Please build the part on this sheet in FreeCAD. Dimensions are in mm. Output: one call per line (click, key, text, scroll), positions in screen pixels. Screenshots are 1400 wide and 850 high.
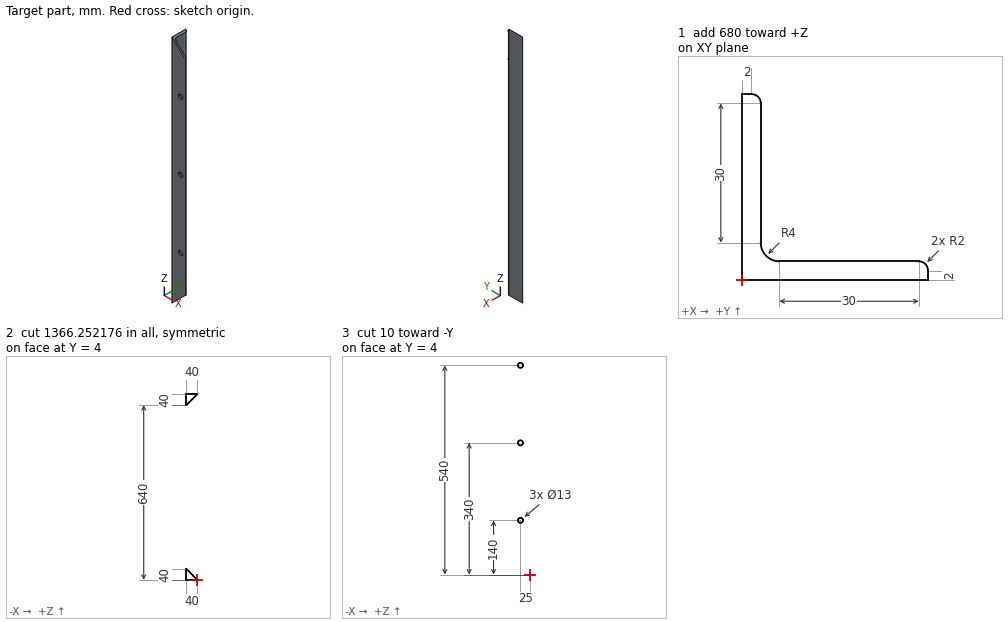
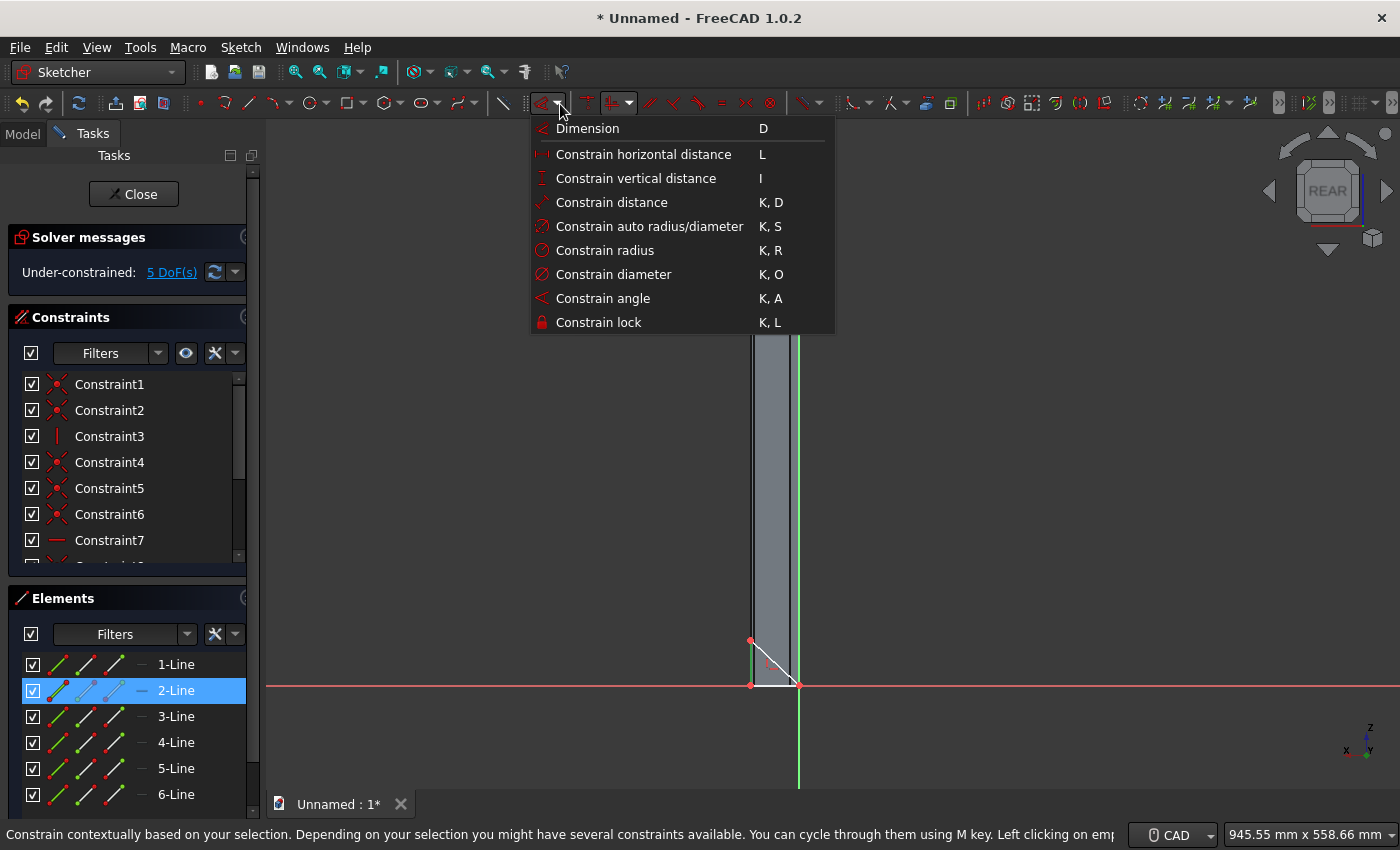
click(683, 178)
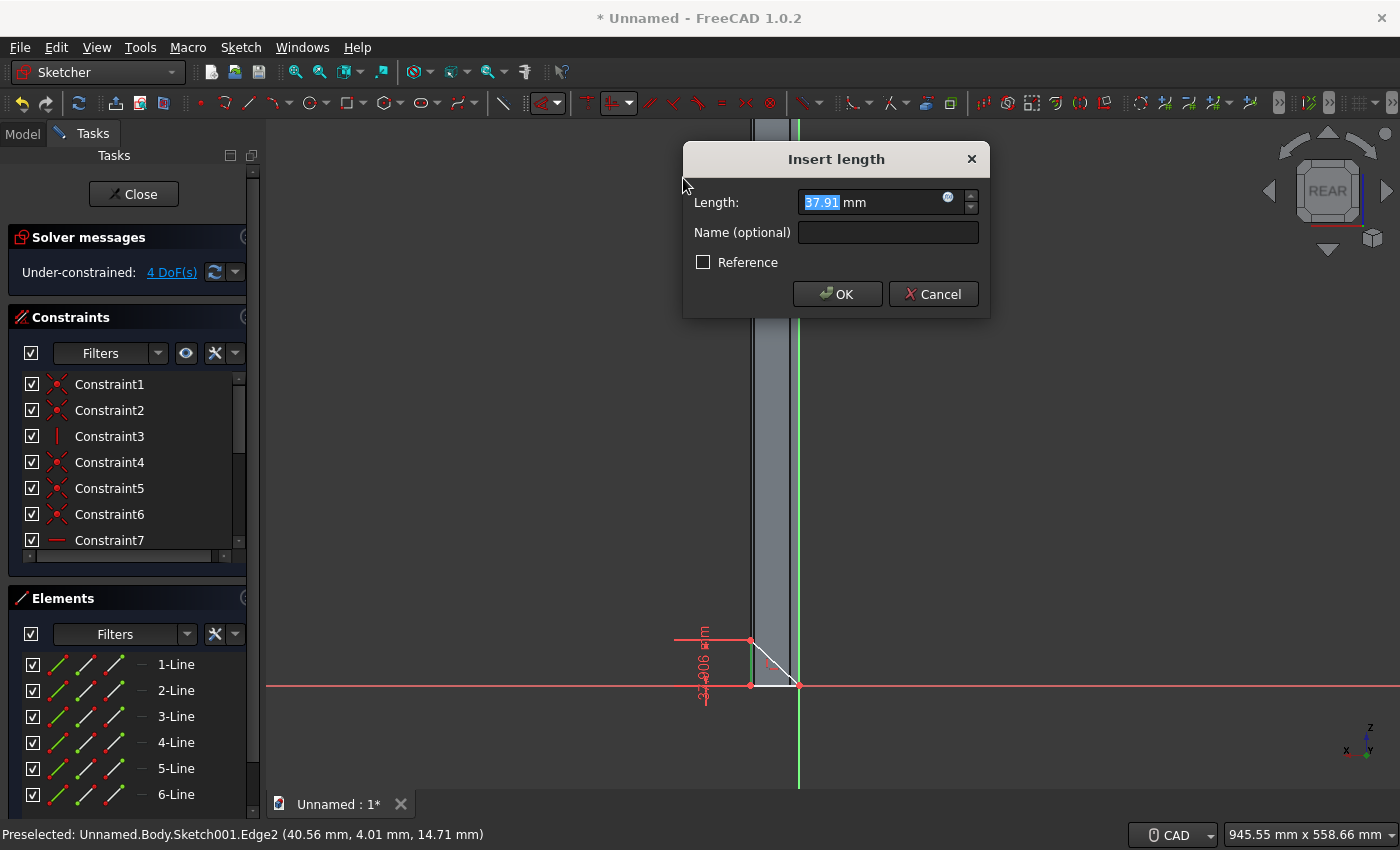
text(40)
key(Return)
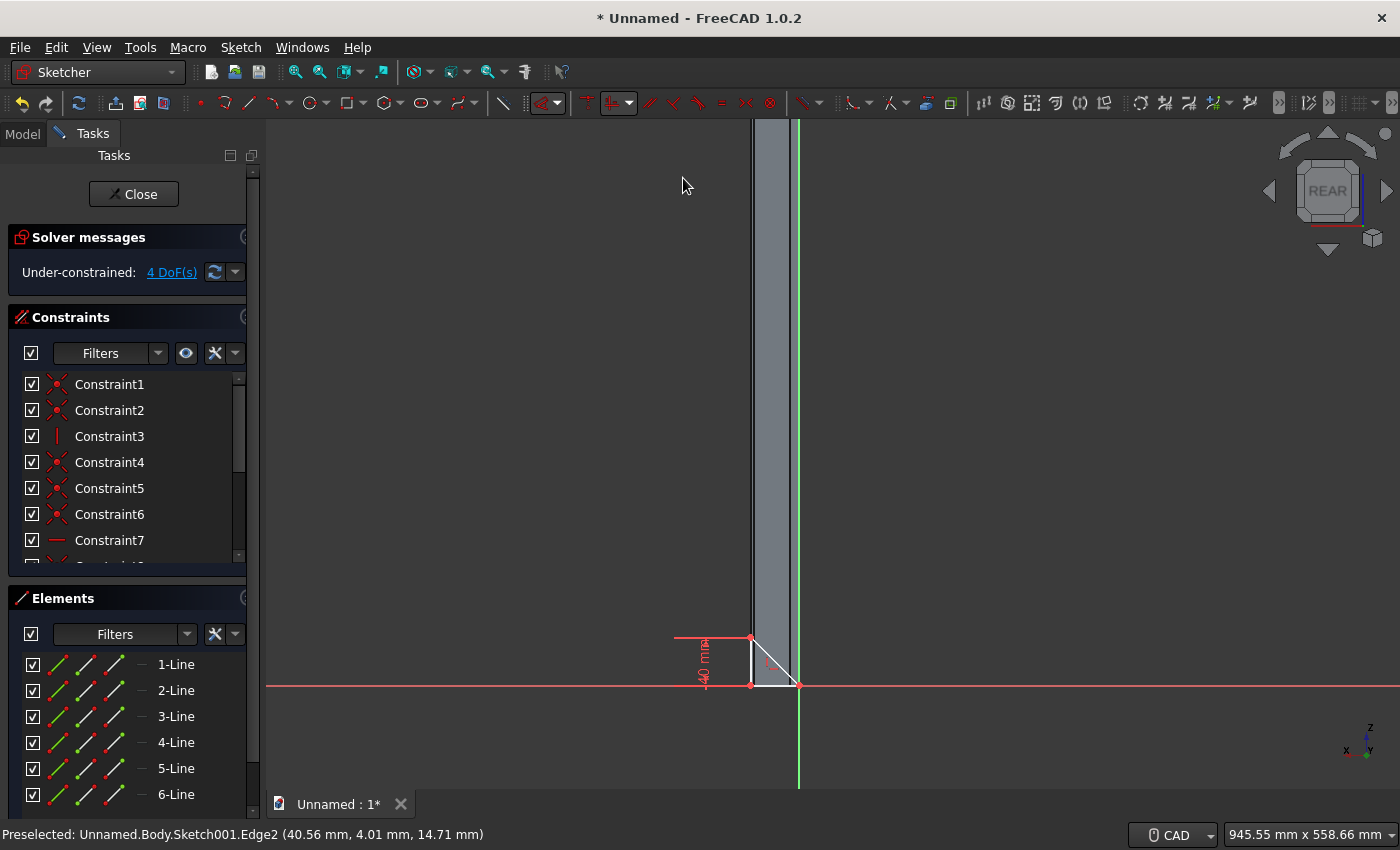
click(765, 686)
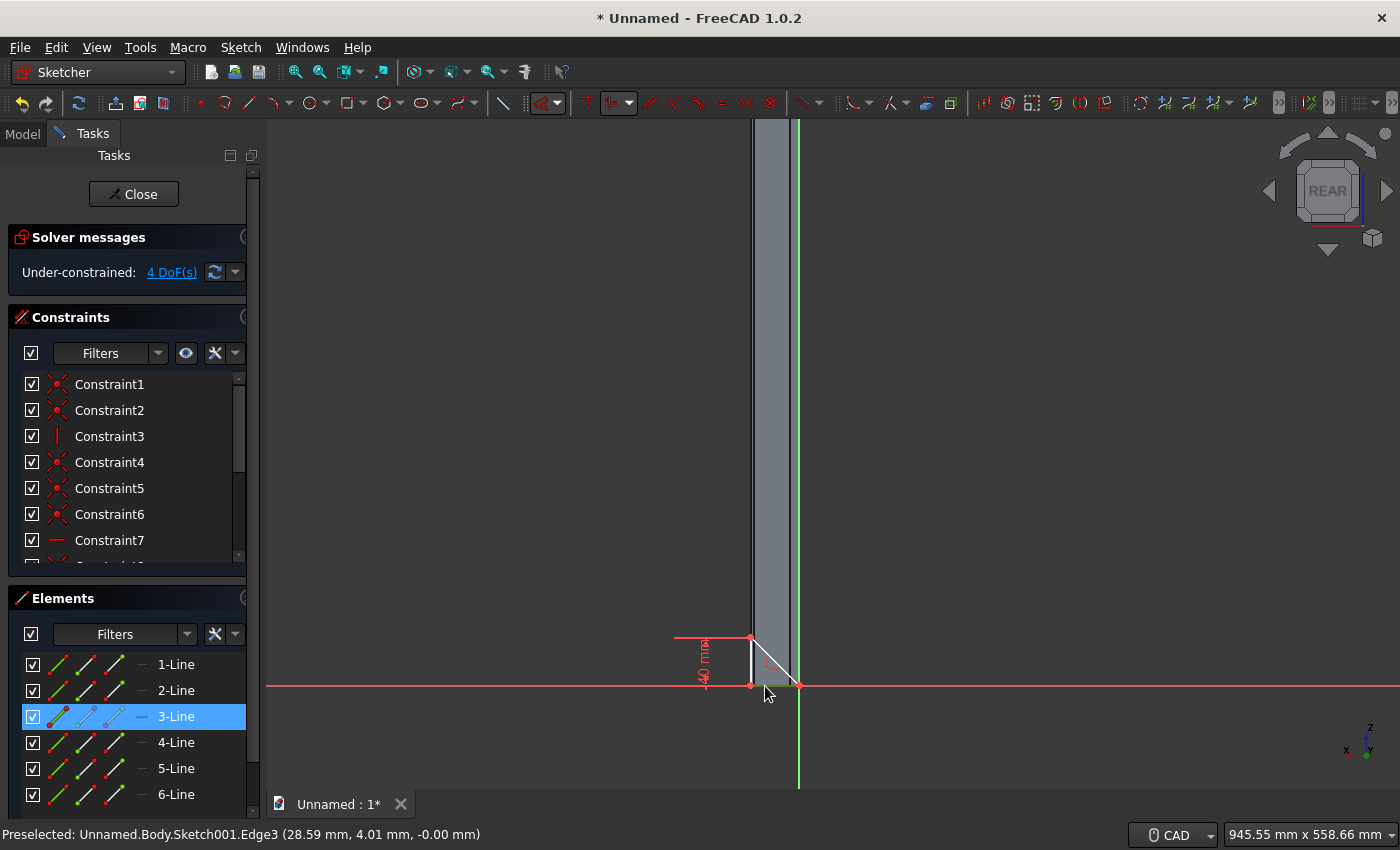
click(560, 104)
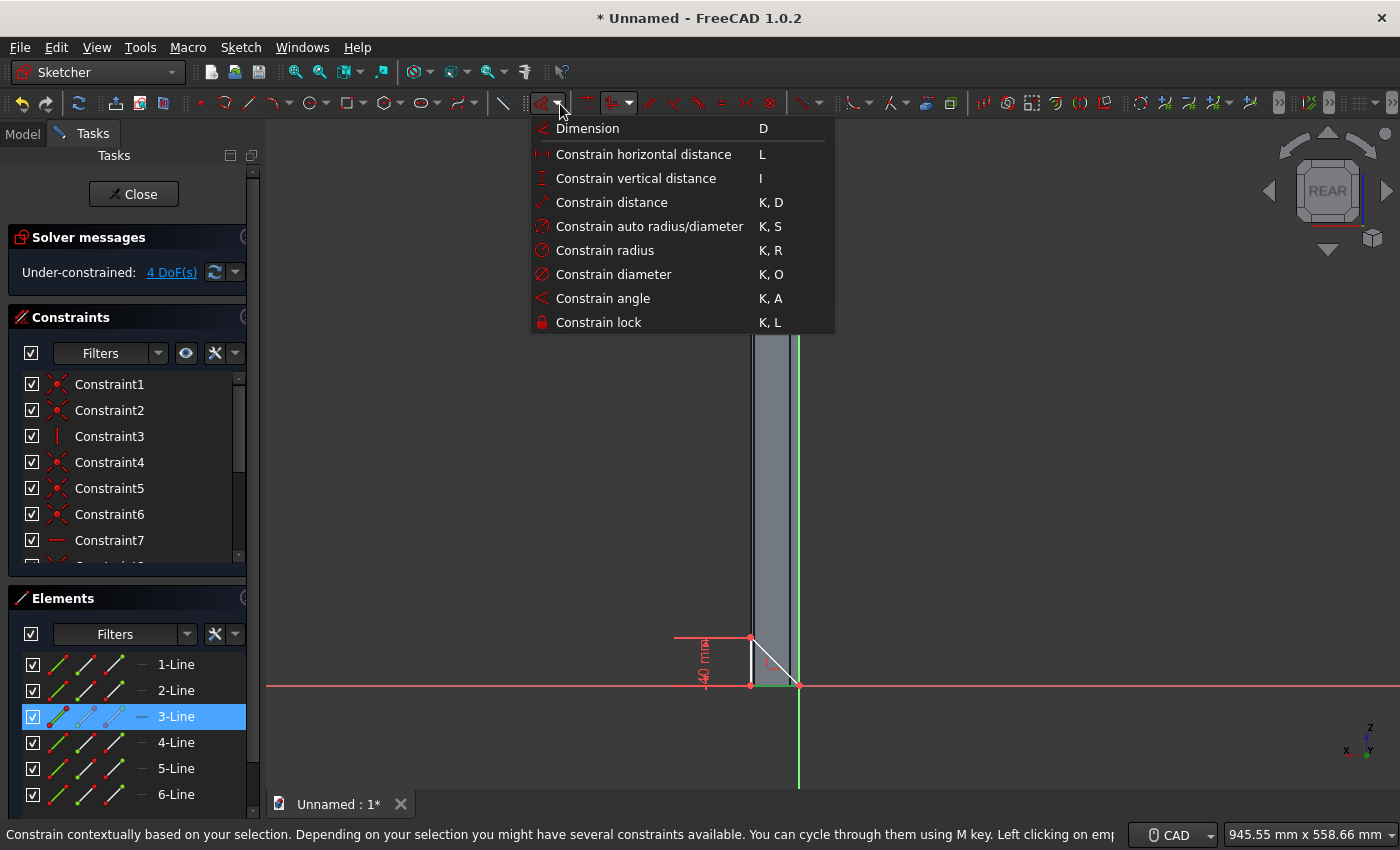
click(683, 154)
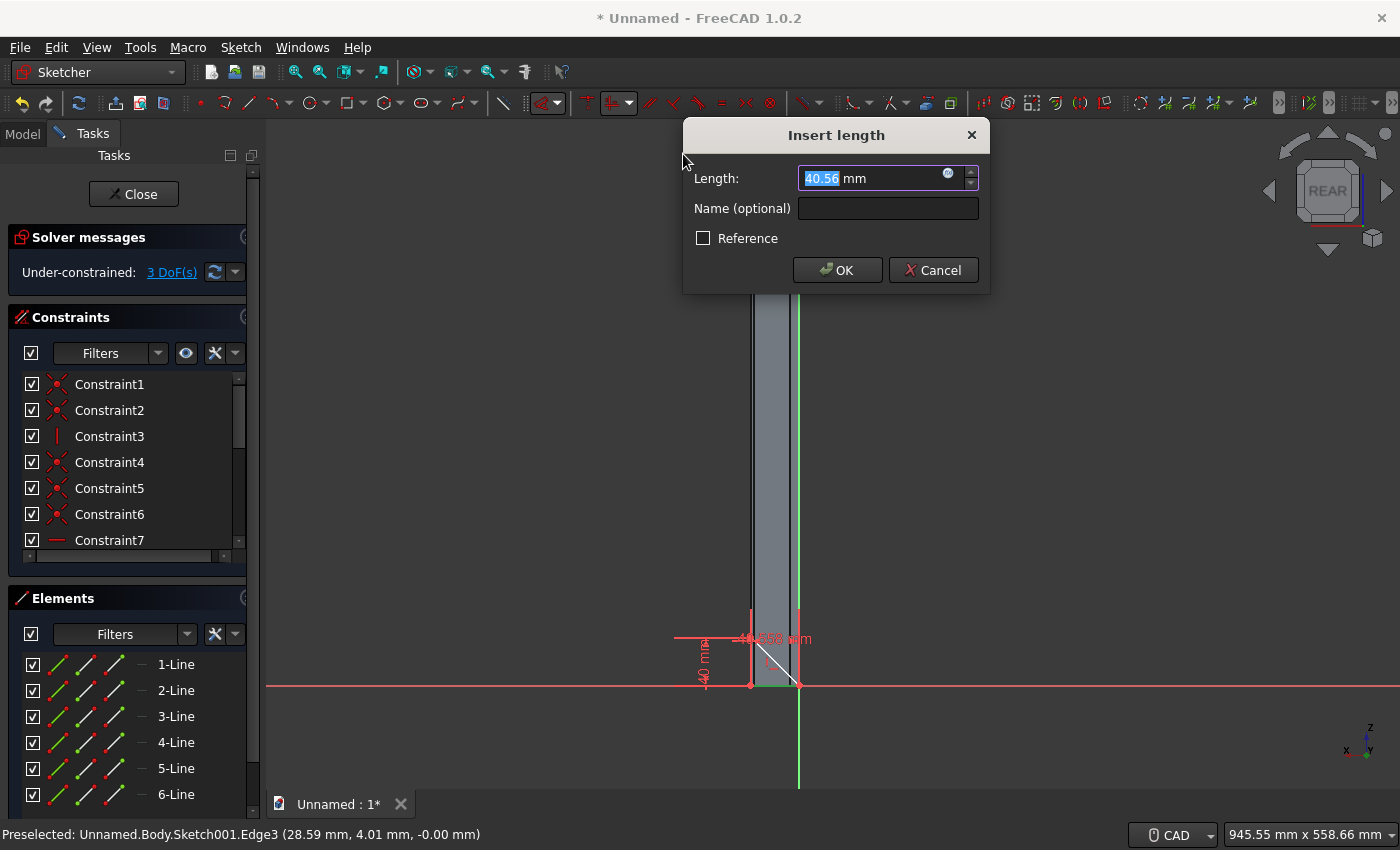
text(40)
key(Return)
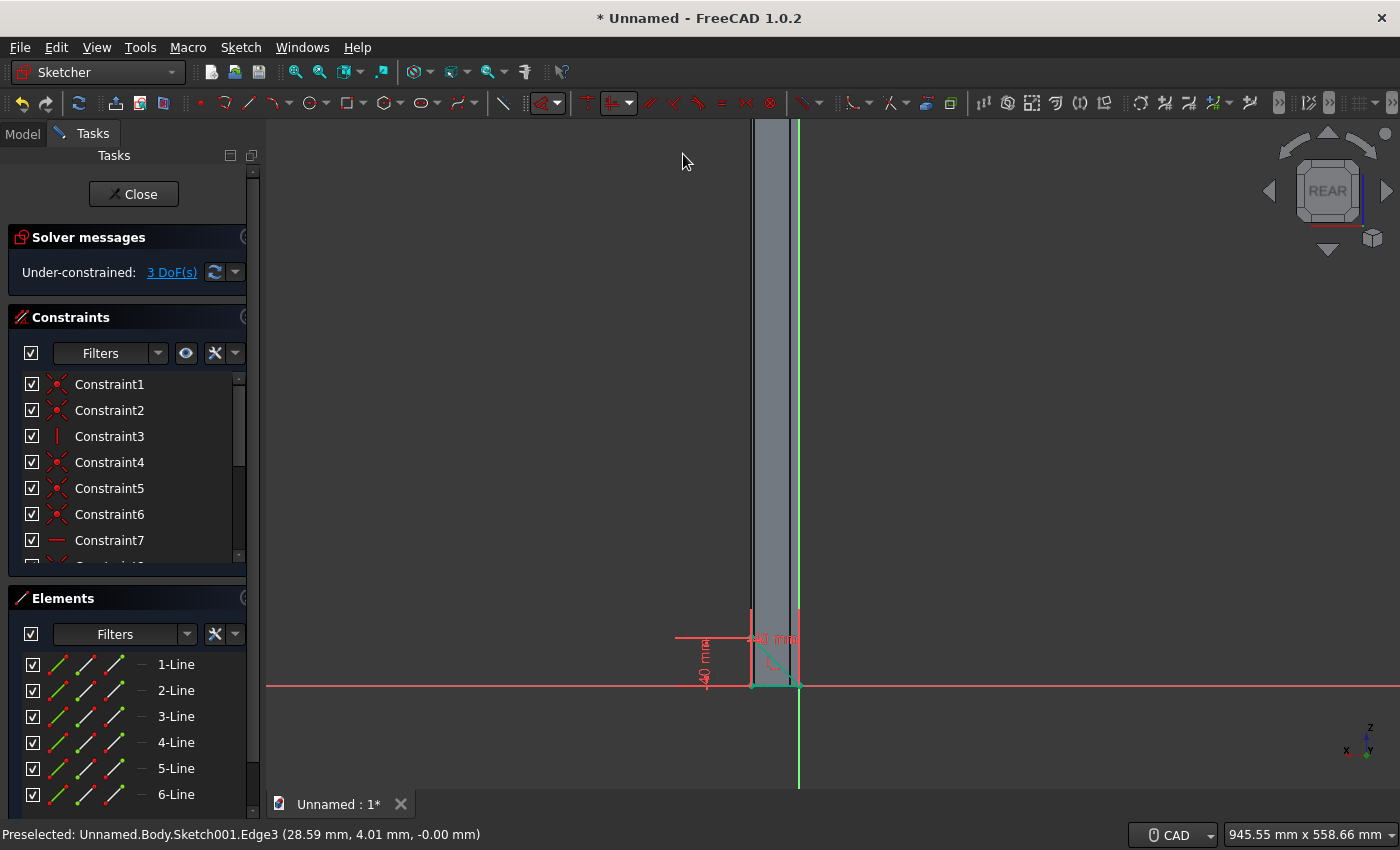
scroll(751, 668, down, 3)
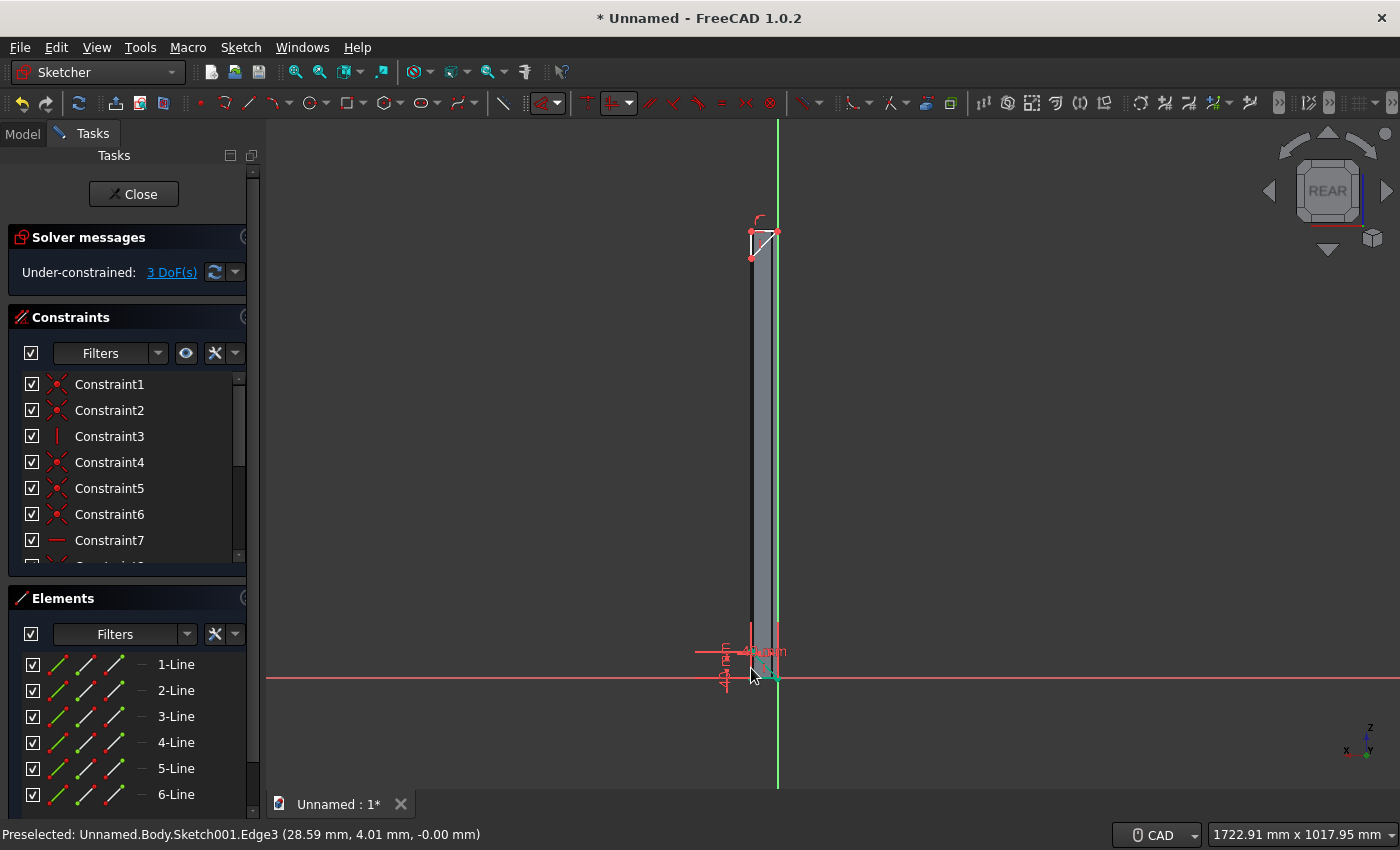
scroll(770, 231, up, 5)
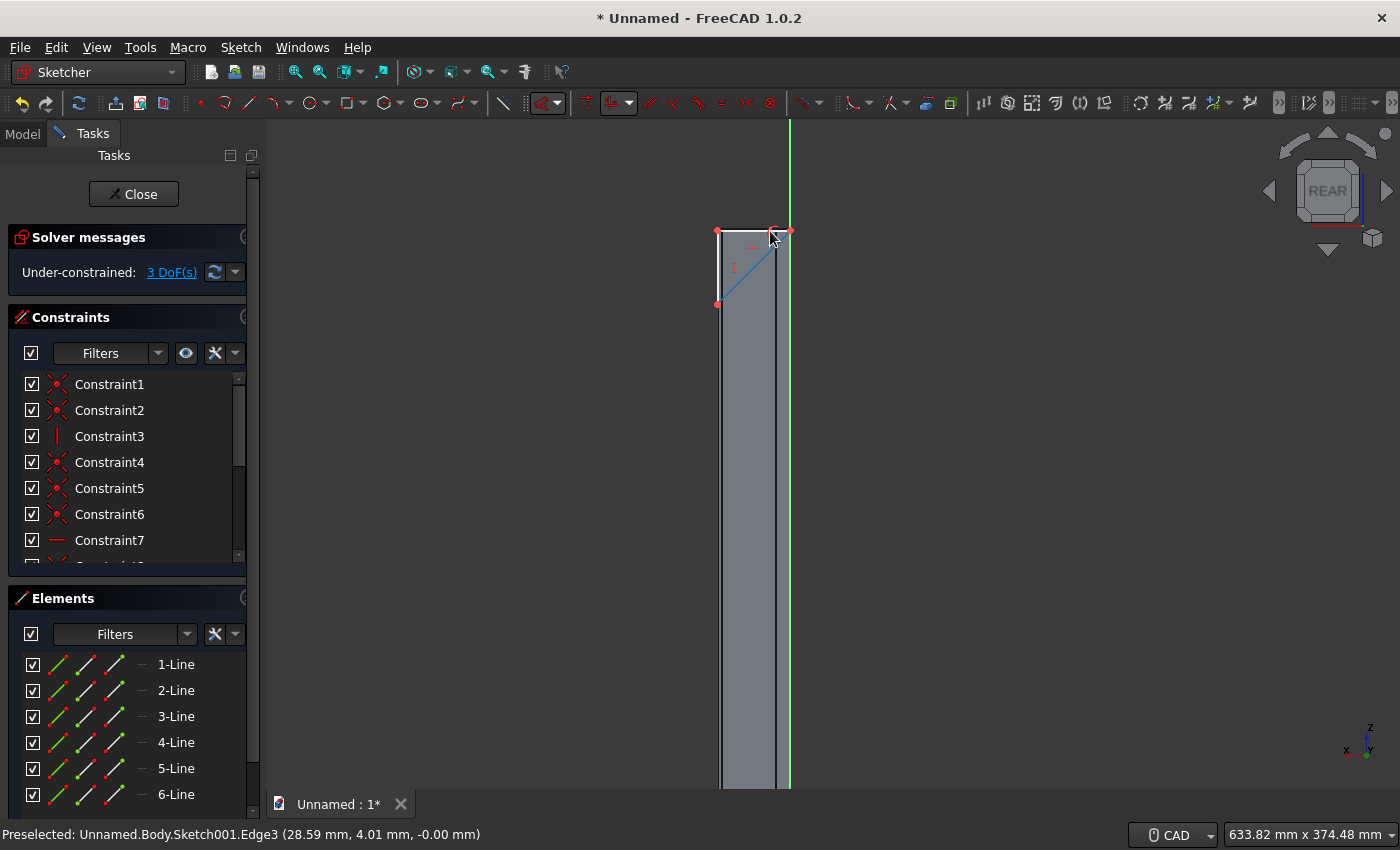
click(739, 231)